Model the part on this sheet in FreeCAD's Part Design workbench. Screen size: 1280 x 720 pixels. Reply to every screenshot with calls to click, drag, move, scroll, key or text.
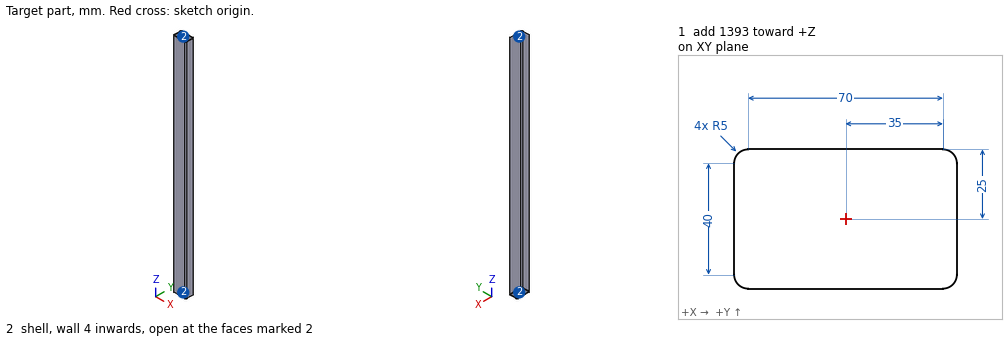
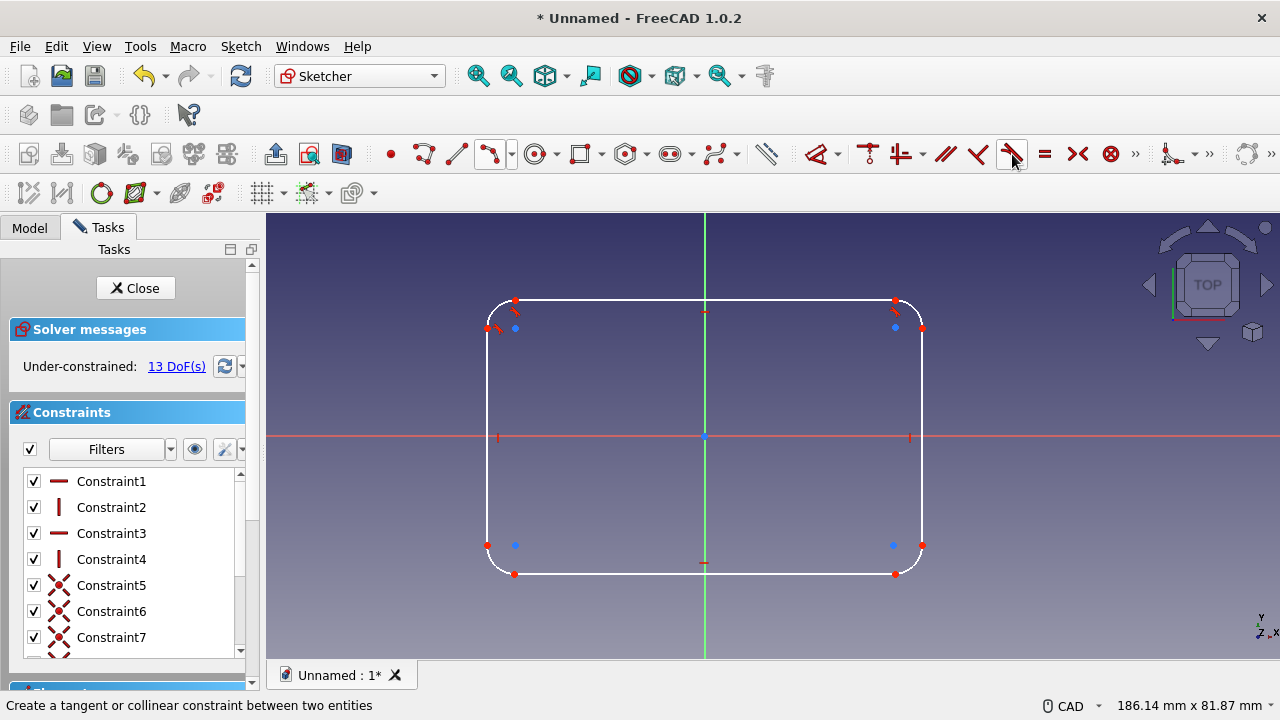
click(487, 394)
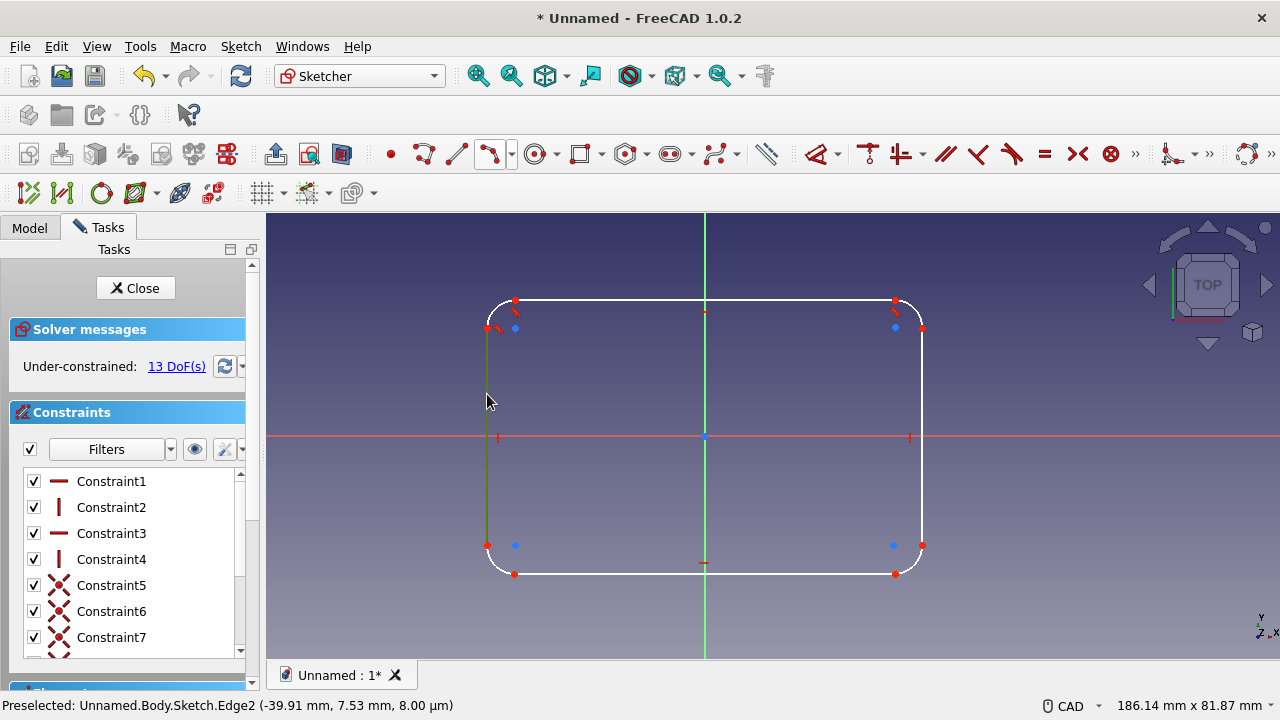
click(490, 558)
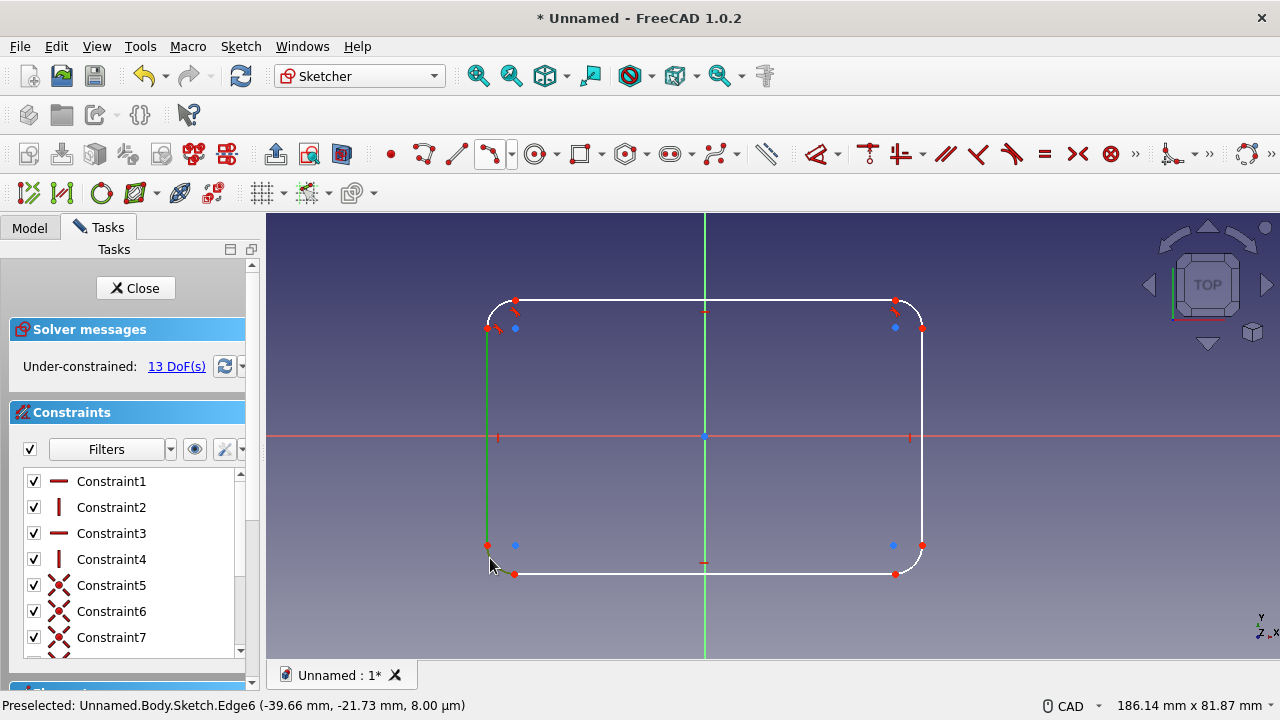
click(1012, 154)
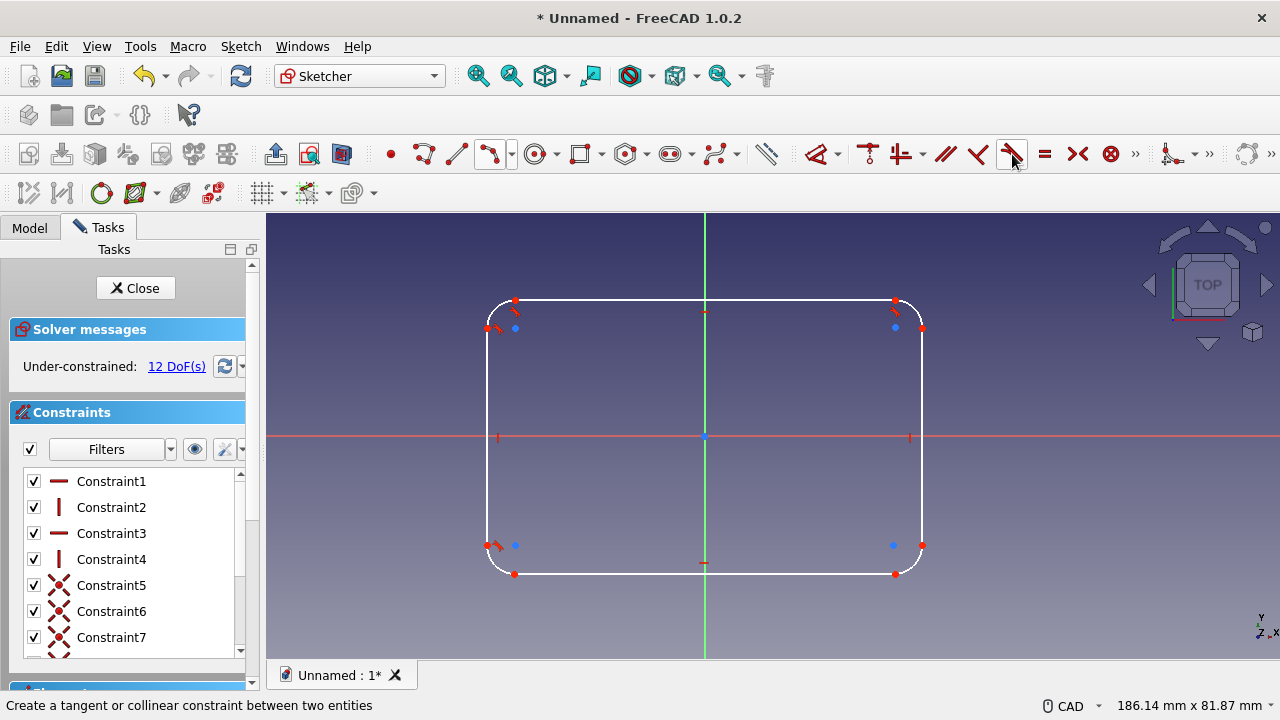
click(628, 574)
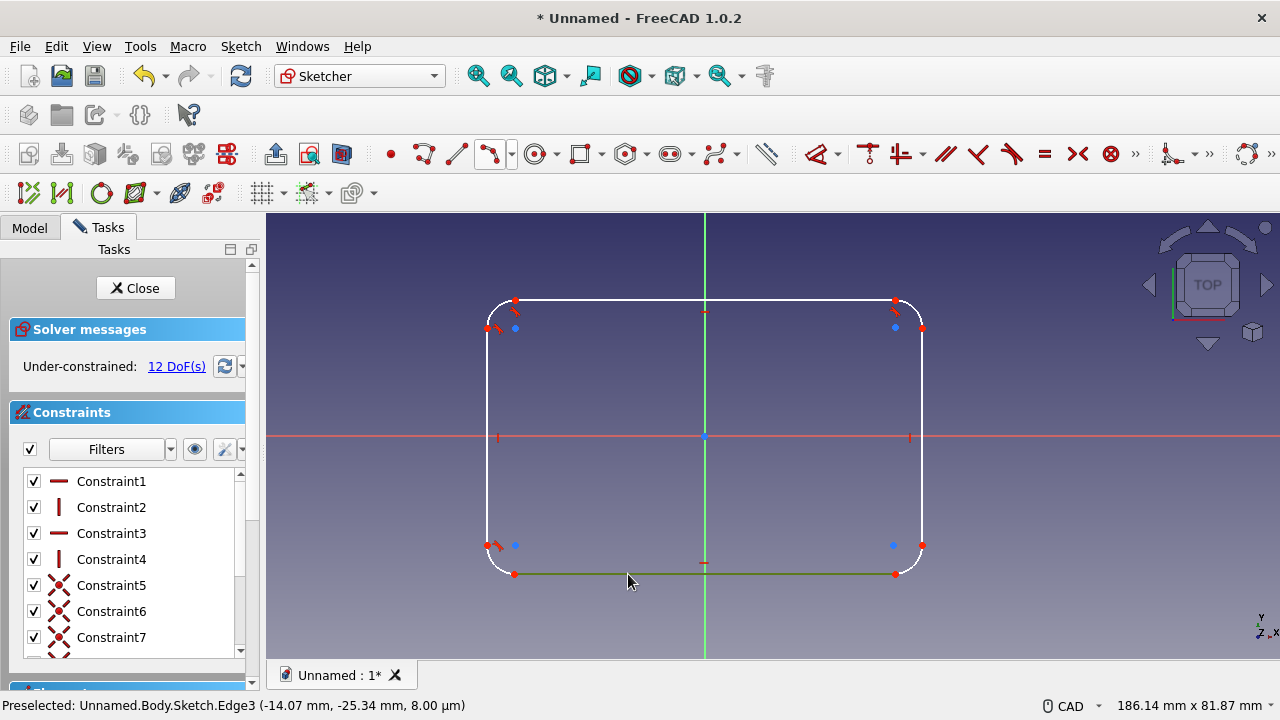
click(490, 558)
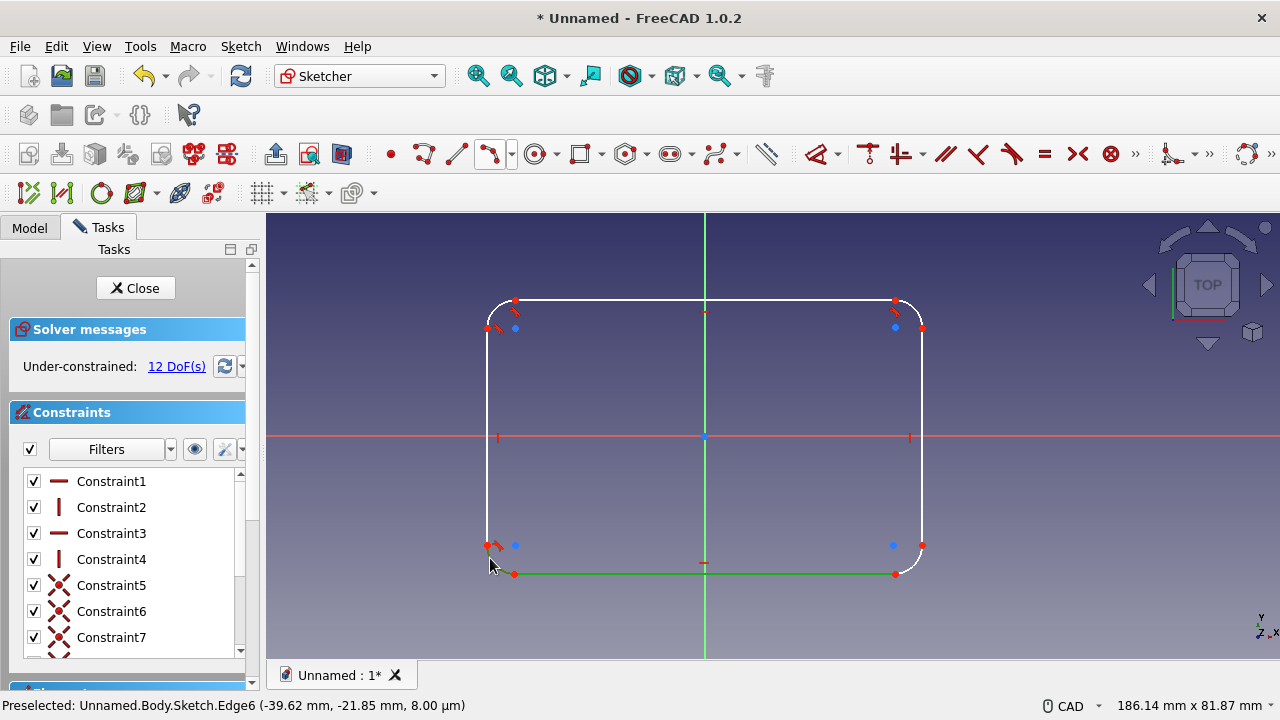
click(1012, 154)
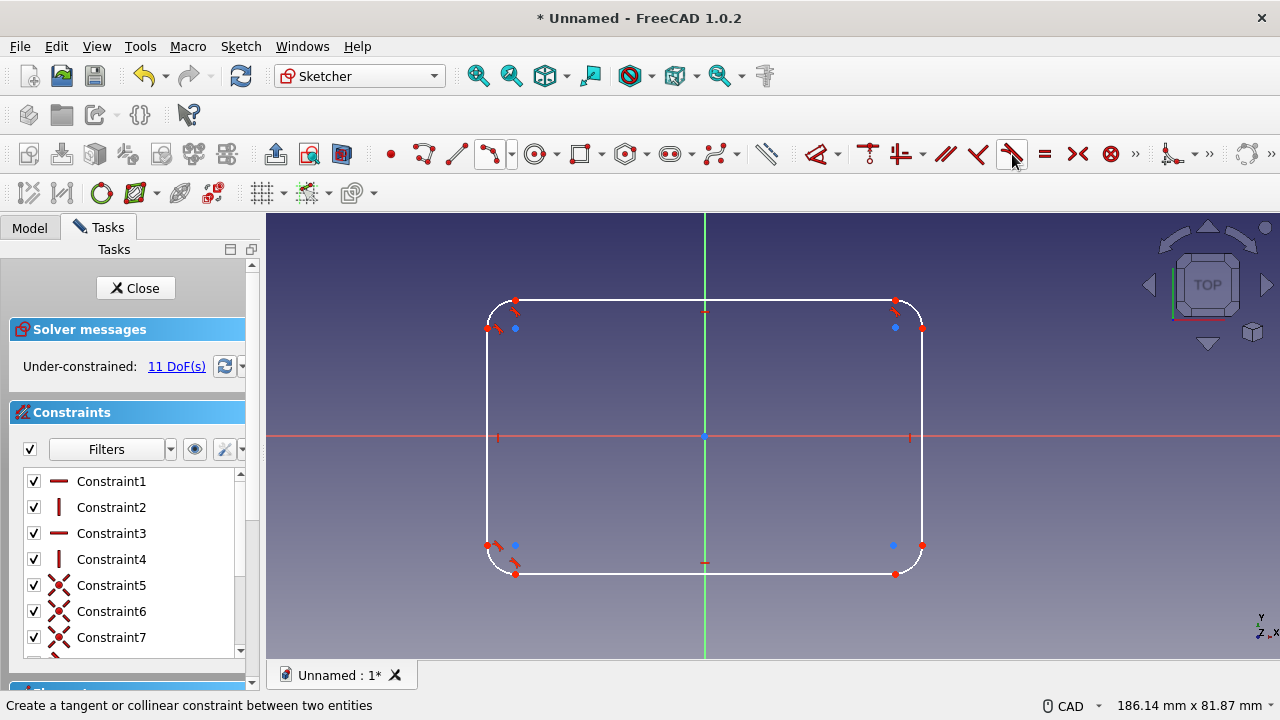
click(629, 574)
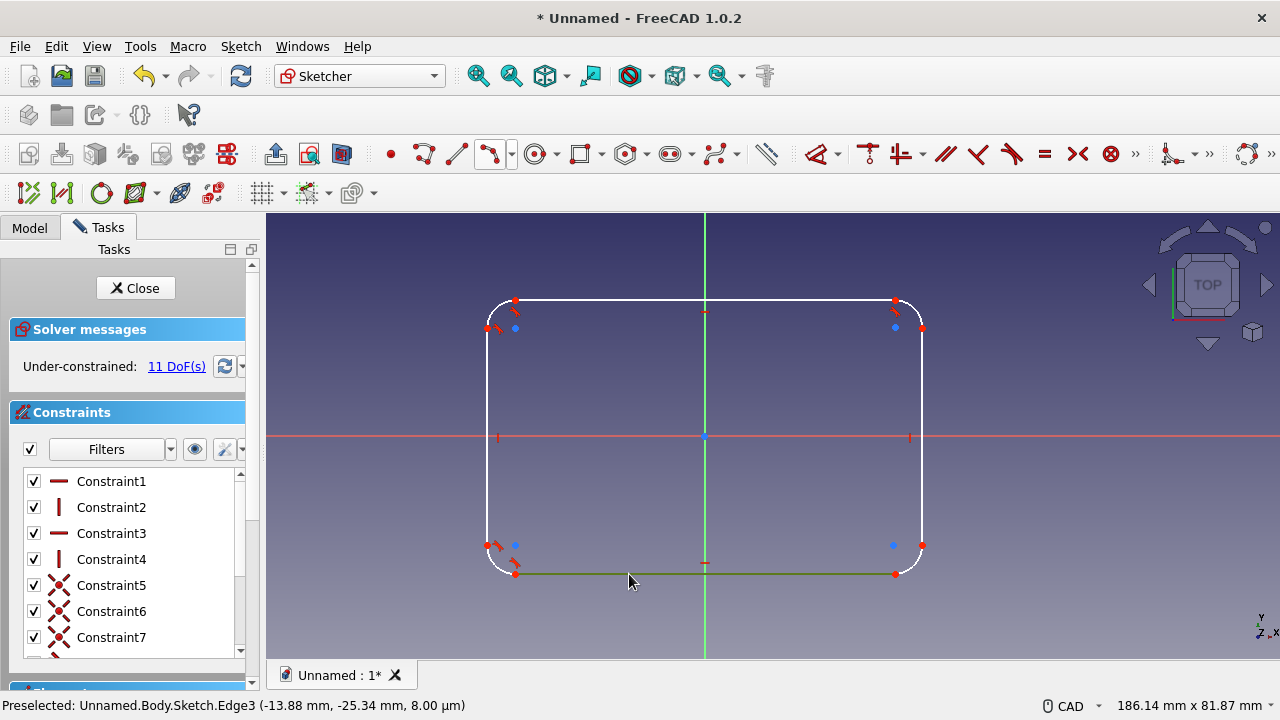
click(907, 570)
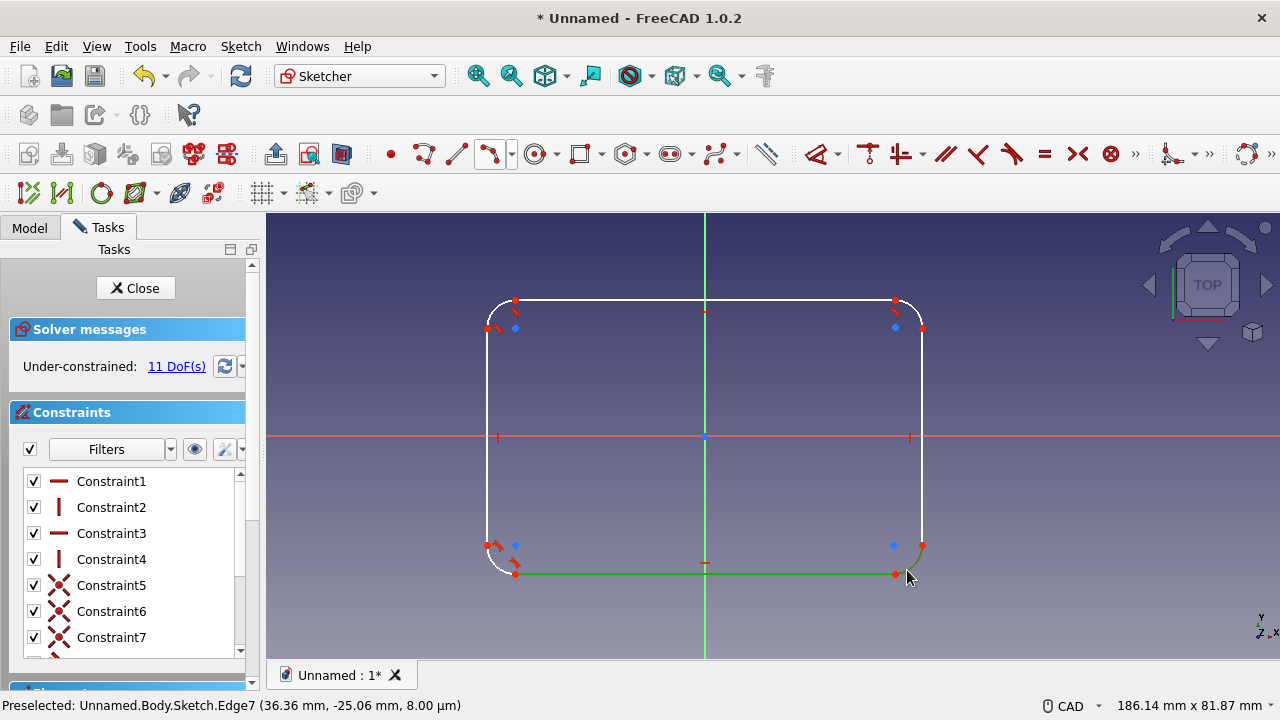
click(1012, 154)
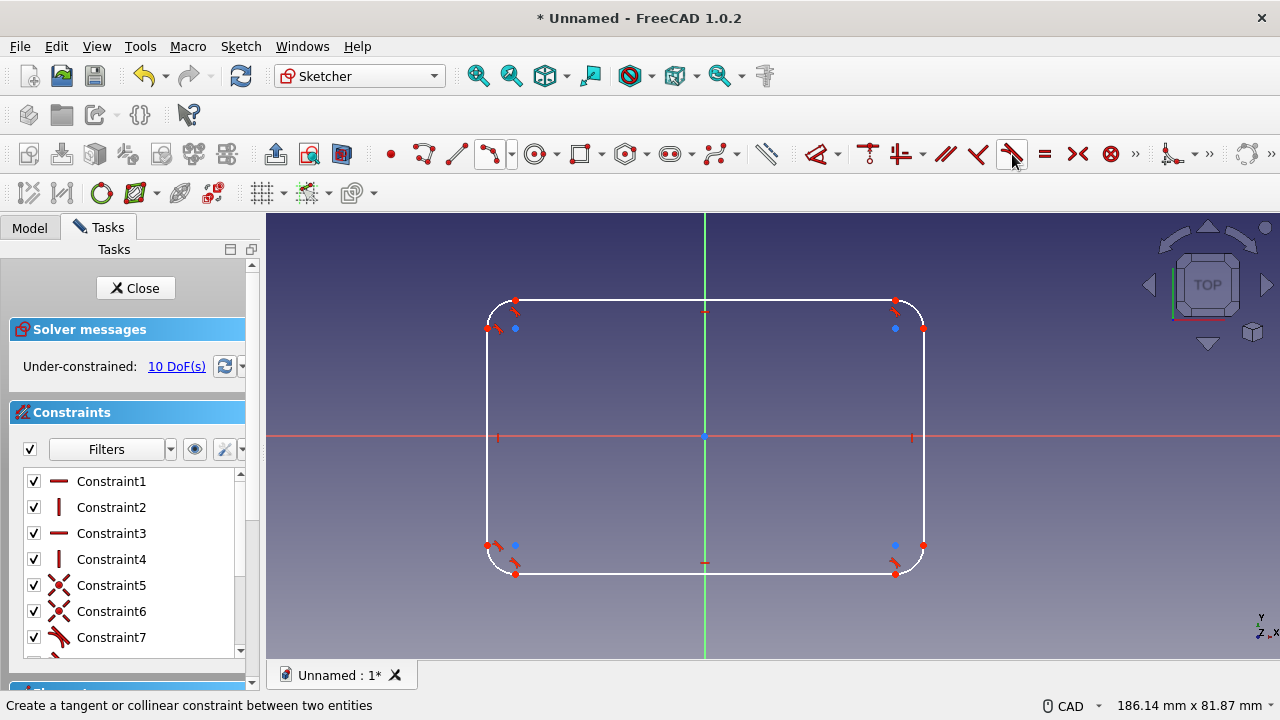
click(924, 481)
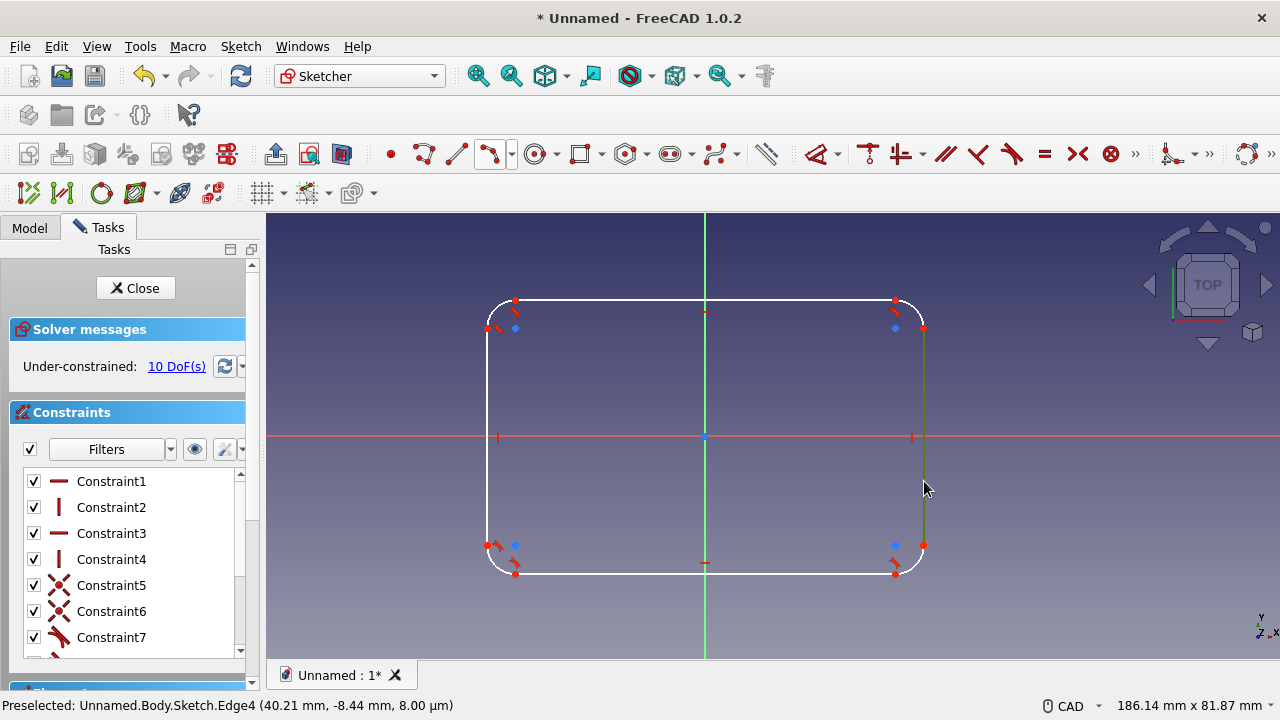
click(908, 571)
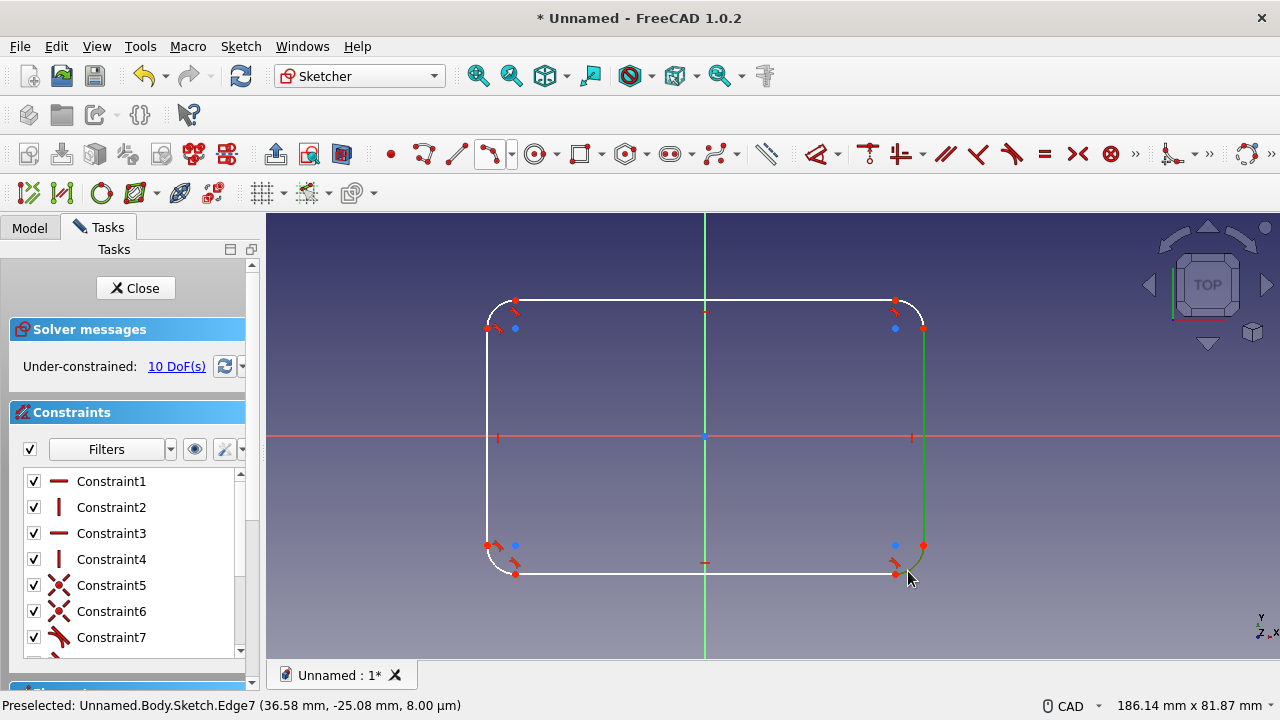
click(1012, 154)